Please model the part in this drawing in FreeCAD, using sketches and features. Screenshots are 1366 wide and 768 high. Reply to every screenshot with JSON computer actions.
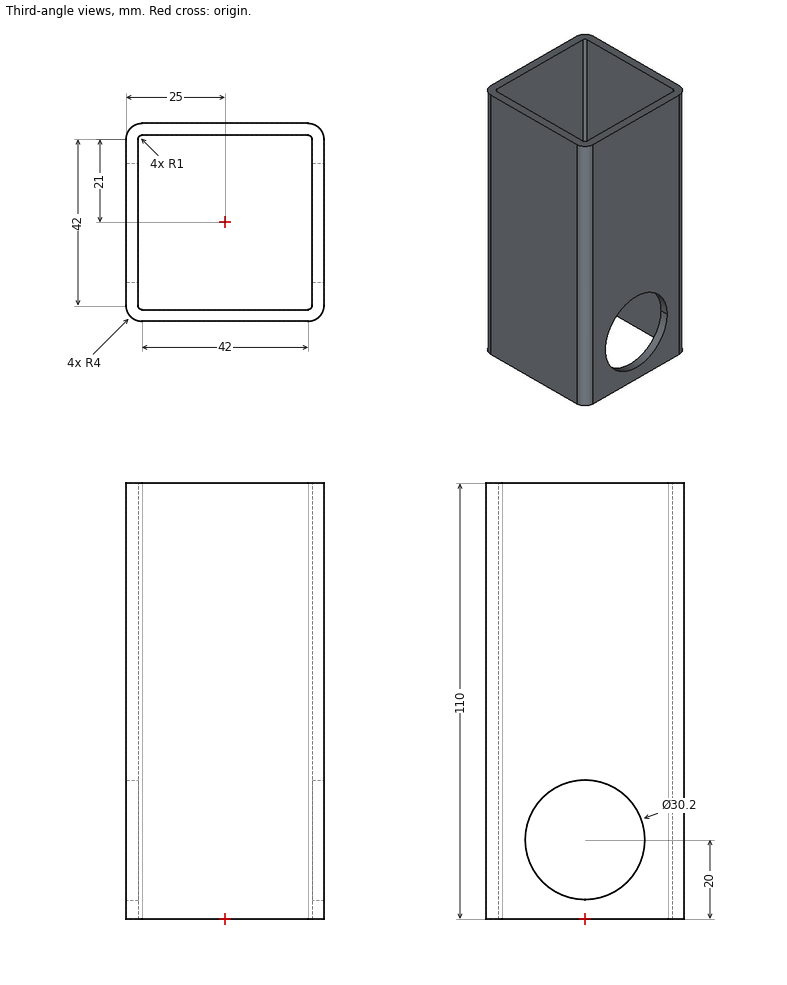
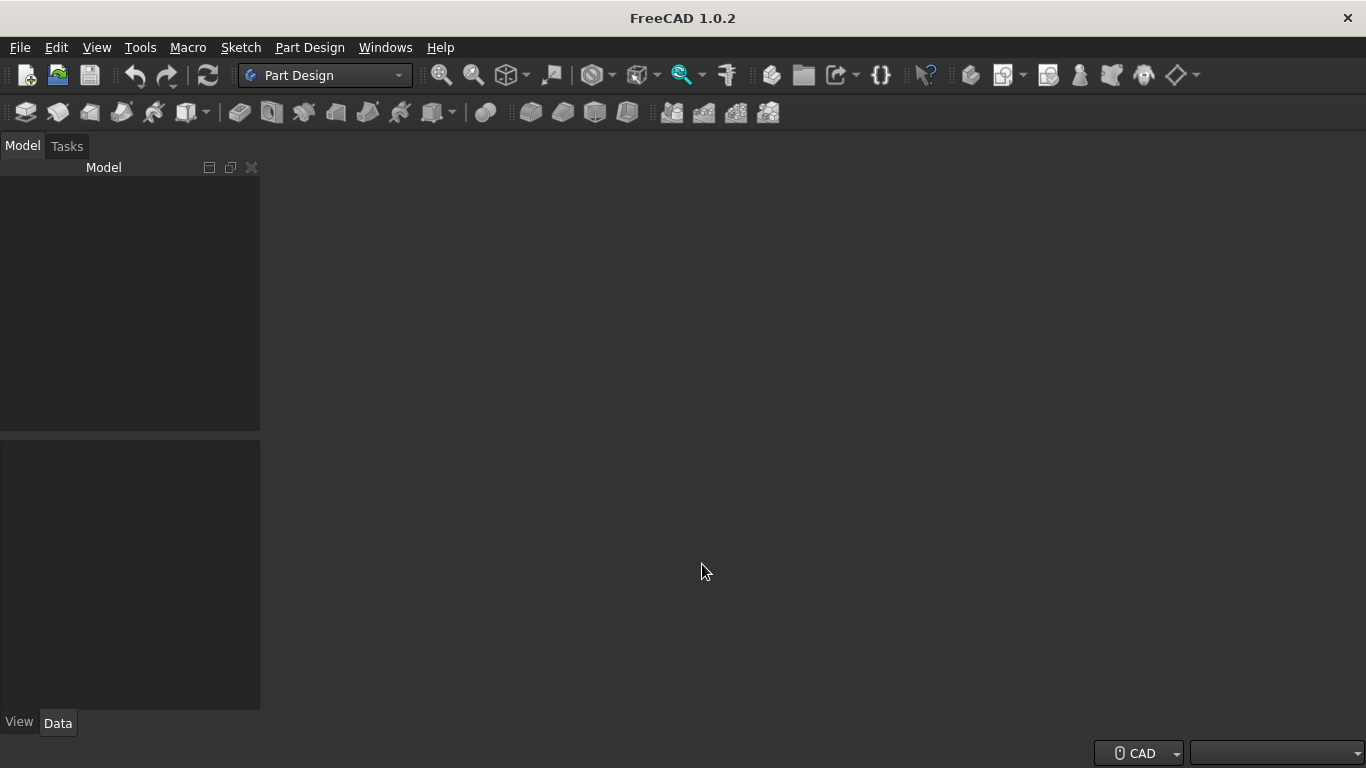
{"action": "left_click", "coordinate": [26, 76]}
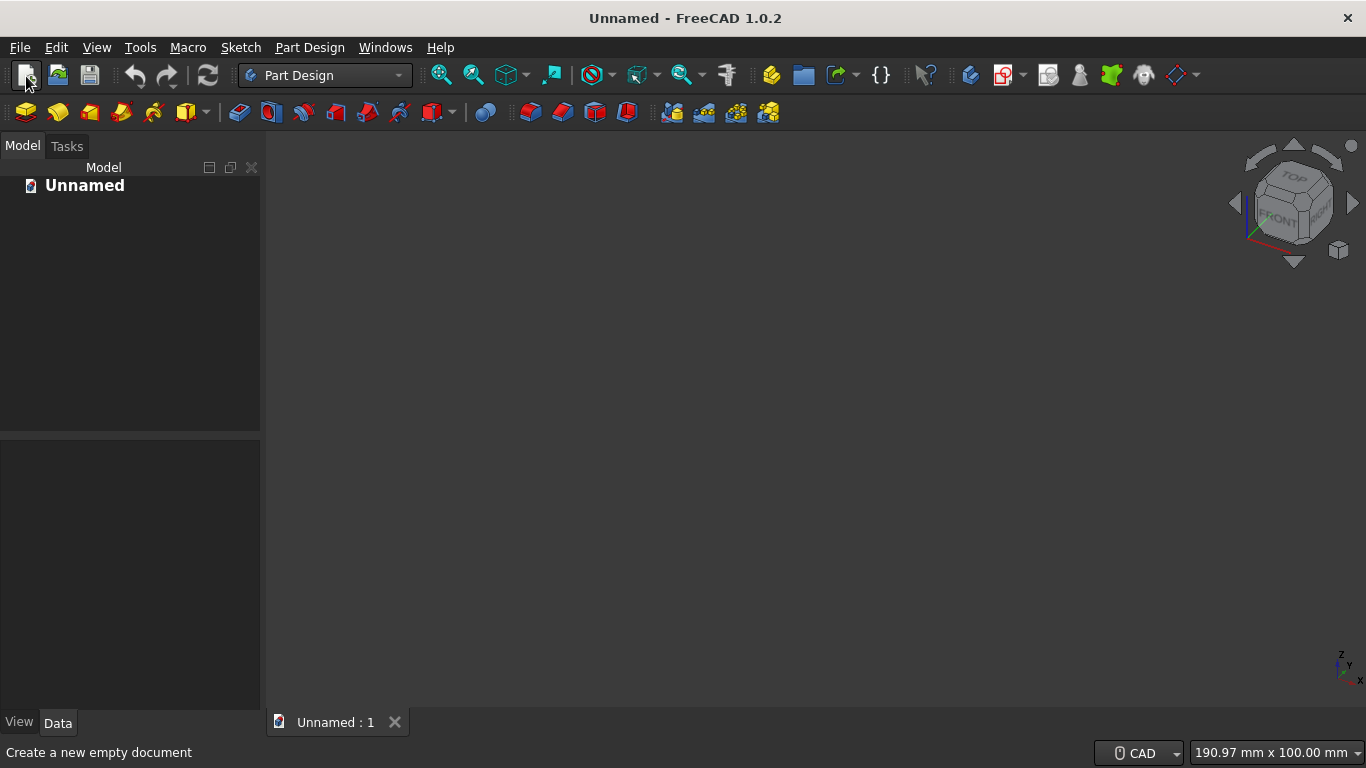
{"action": "left_click", "coordinate": [1004, 76]}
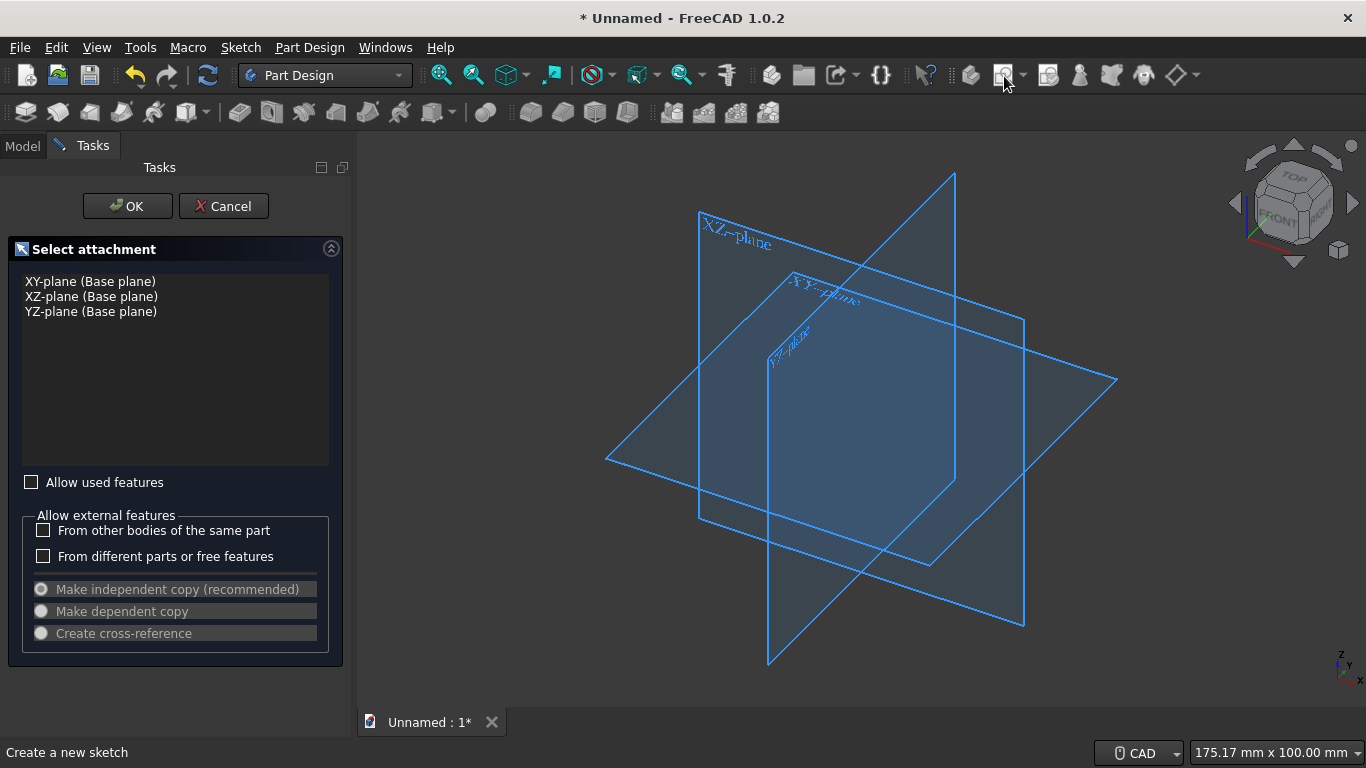
{"action": "left_click", "coordinate": [82, 282]}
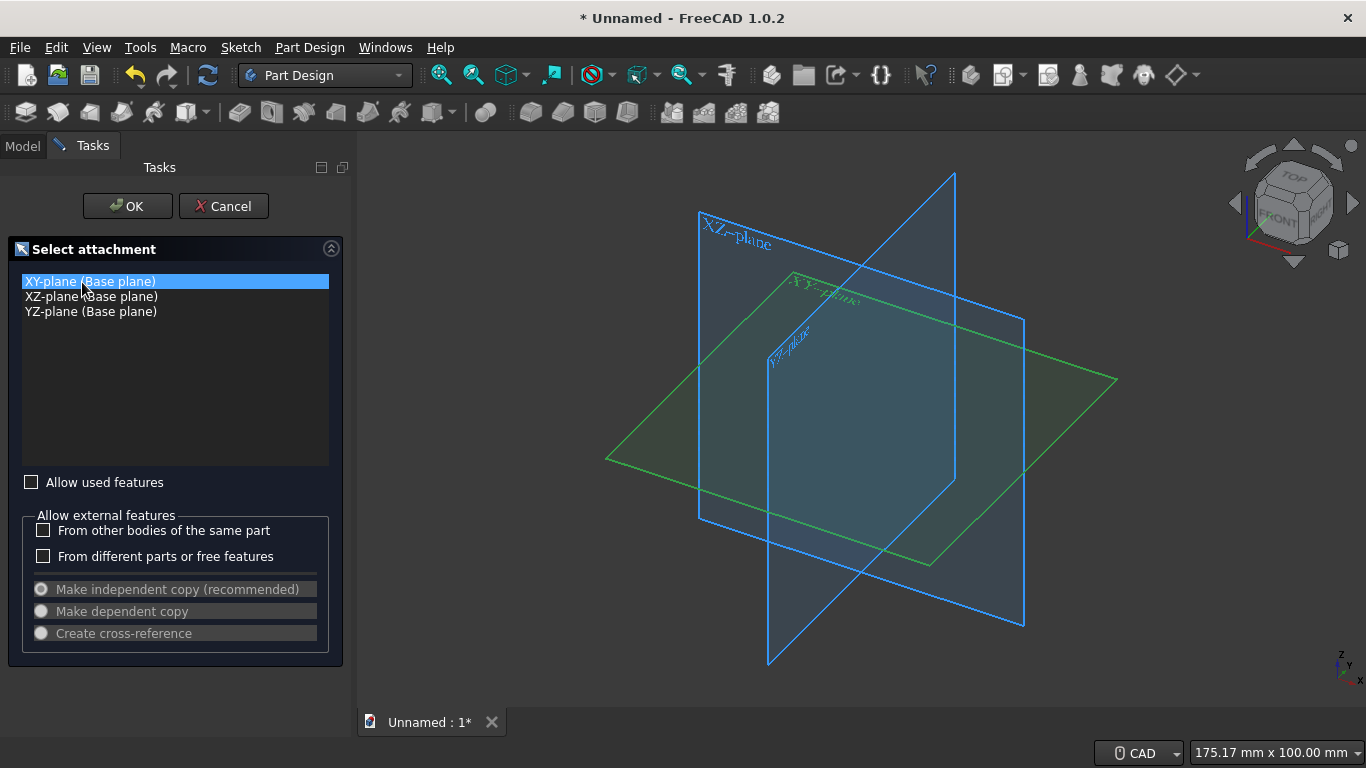
{"action": "left_click", "coordinate": [128, 206]}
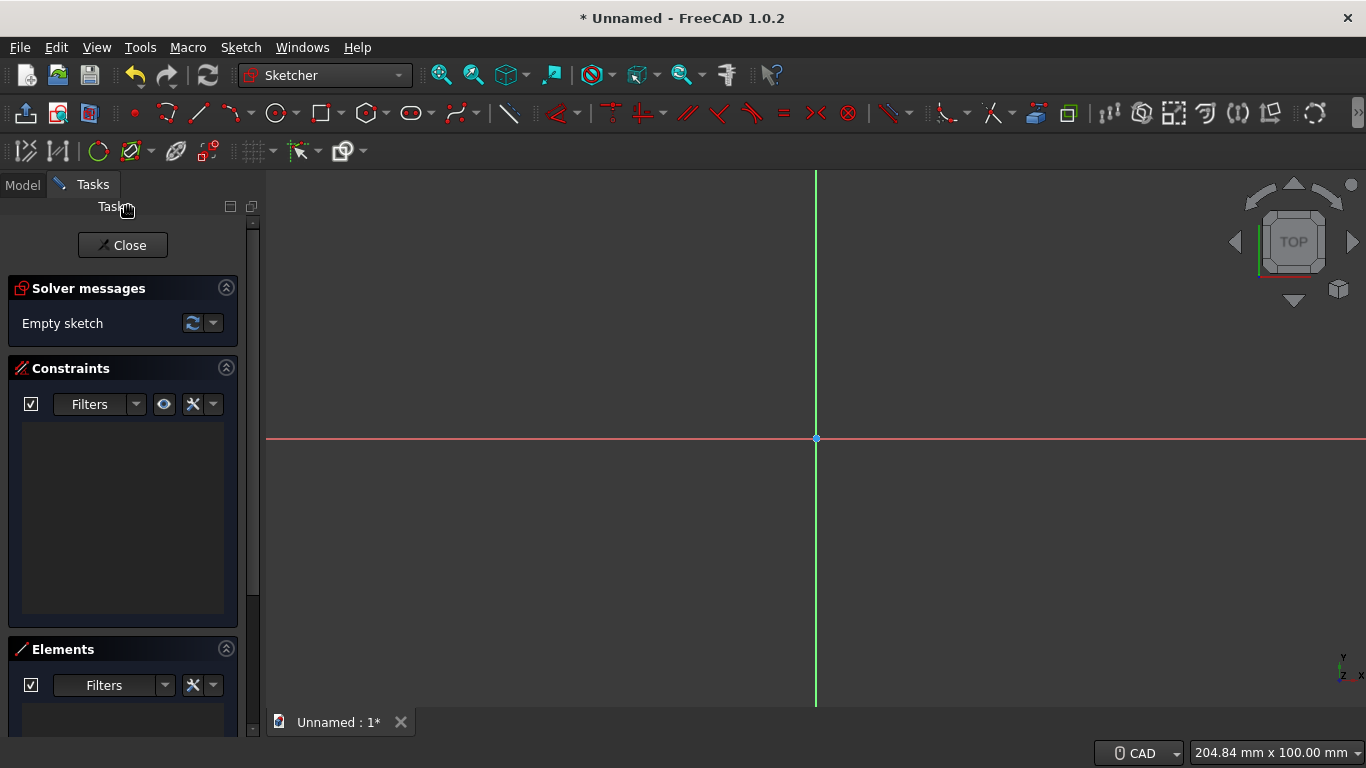
{"action": "left_click", "coordinate": [200, 114]}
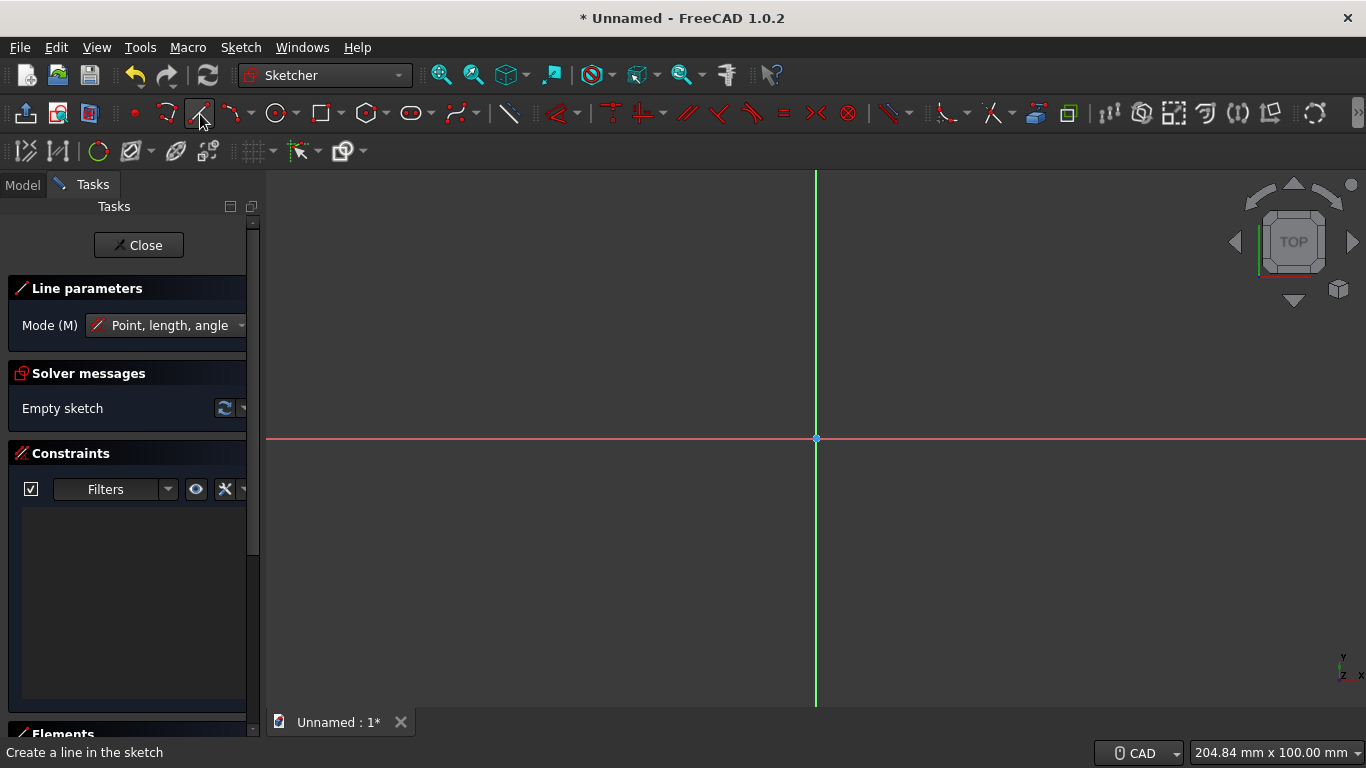
{"action": "left_click", "coordinate": [682, 326]}
{"action": "left_click", "coordinate": [682, 551]}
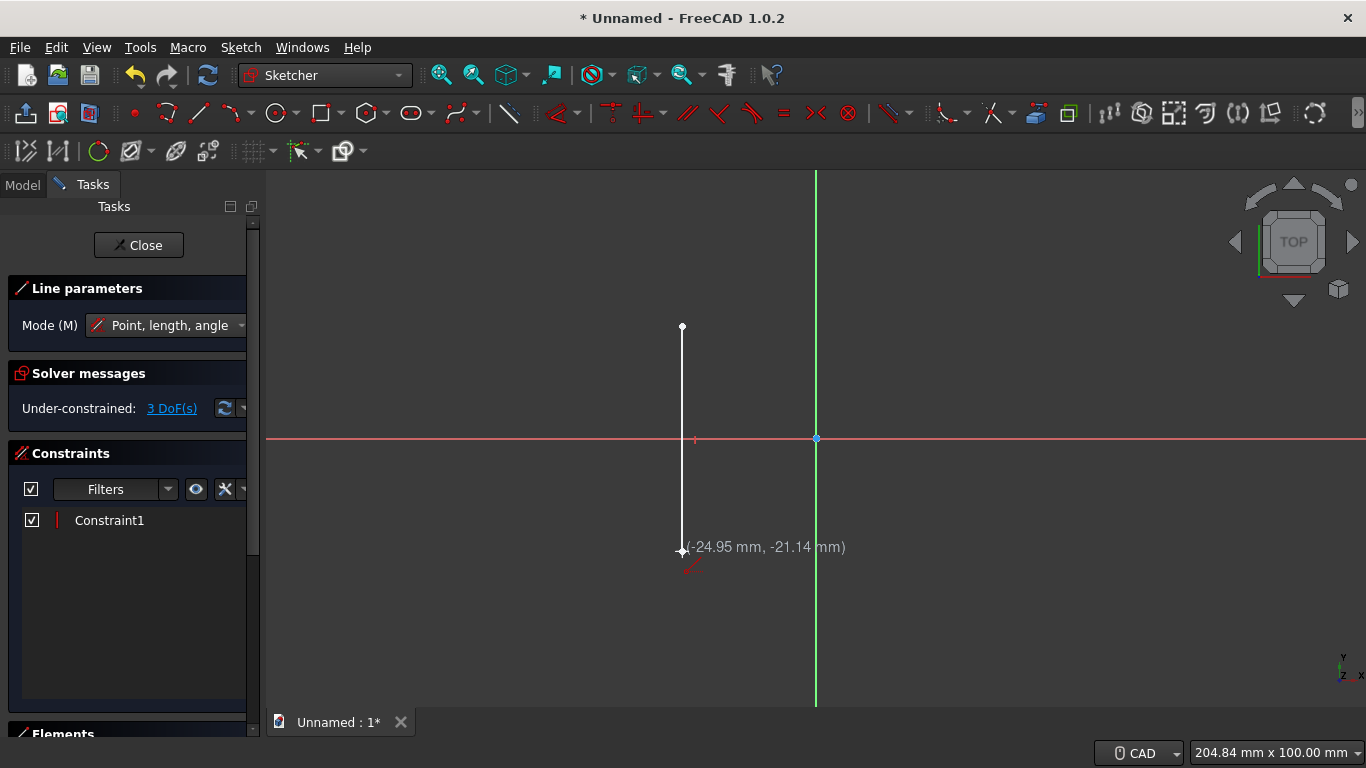
{"action": "left_click", "coordinate": [703, 573]}
{"action": "left_click", "coordinate": [929, 573]}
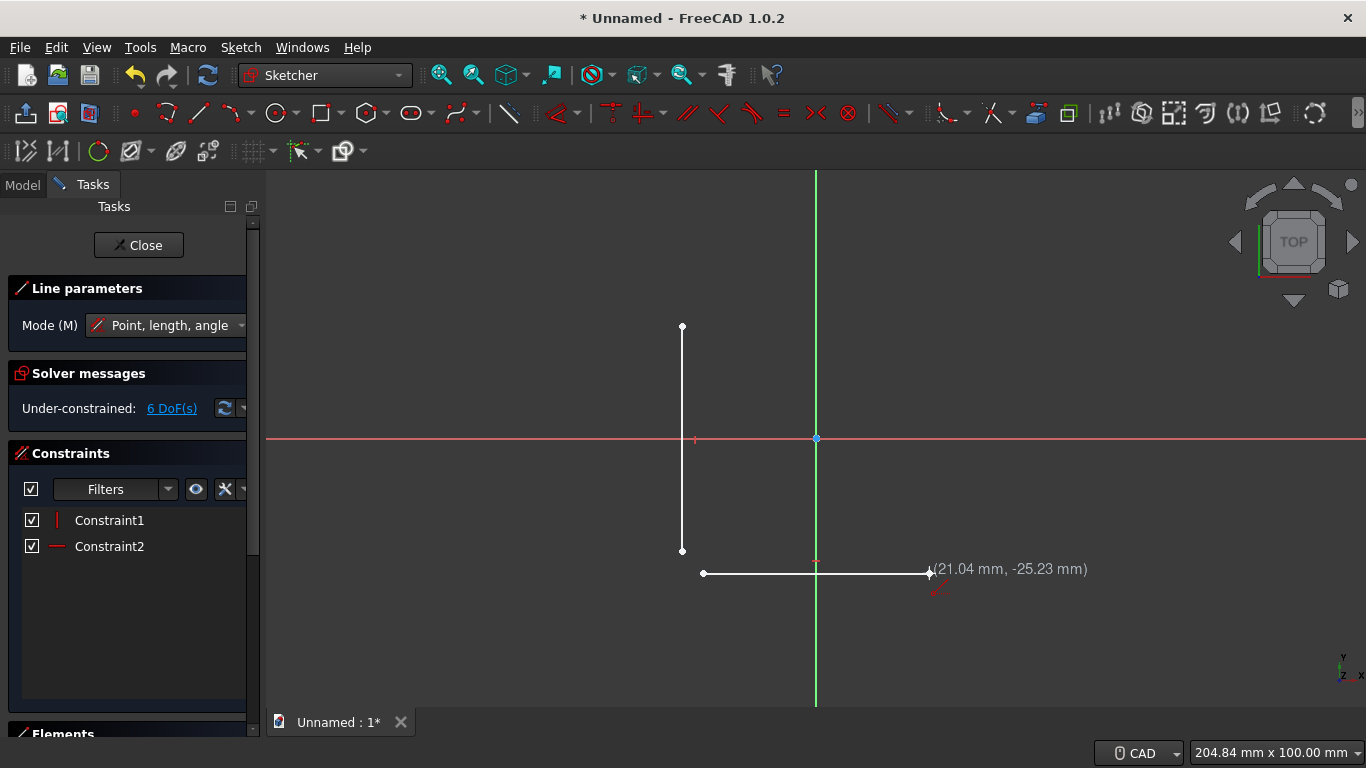
{"action": "left_click", "coordinate": [950, 551]}
{"action": "left_click", "coordinate": [950, 326]}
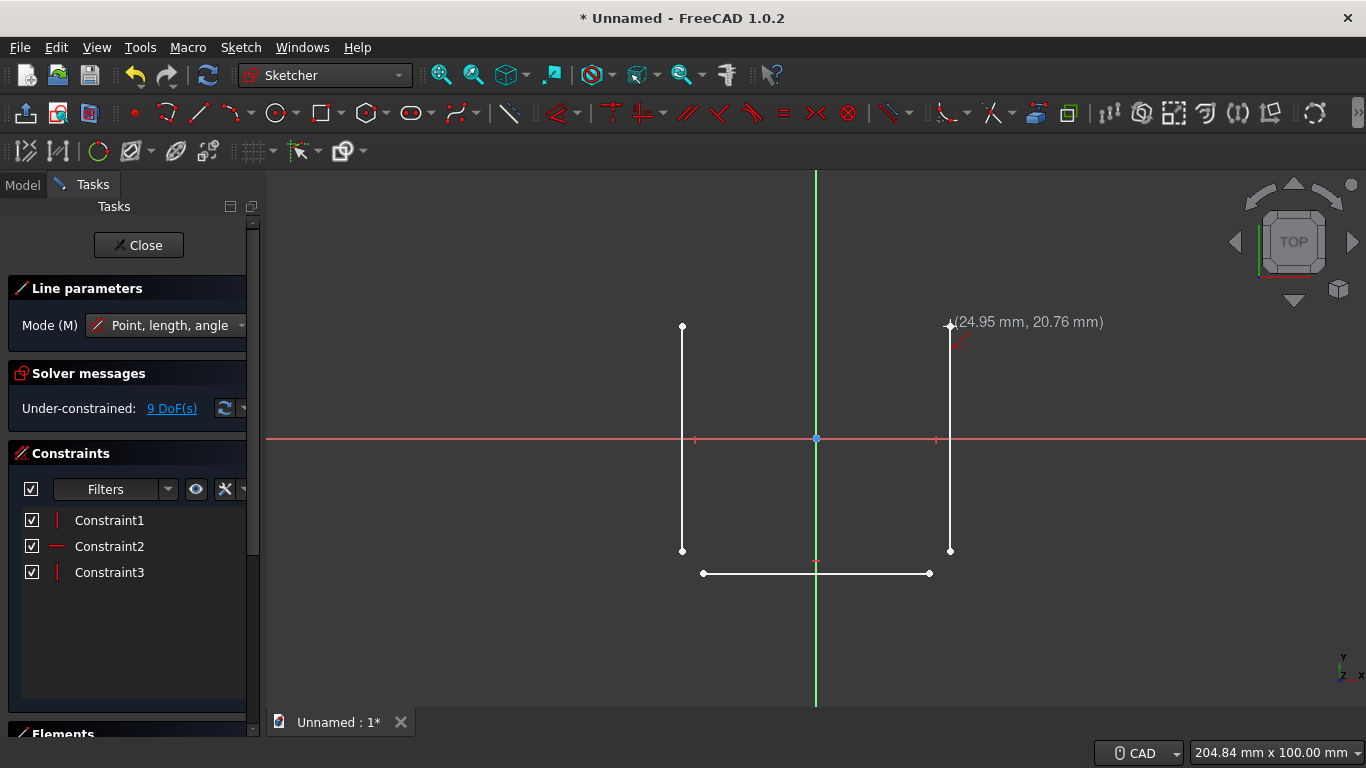
{"action": "left_click", "coordinate": [929, 304]}
{"action": "left_click", "coordinate": [703, 304]}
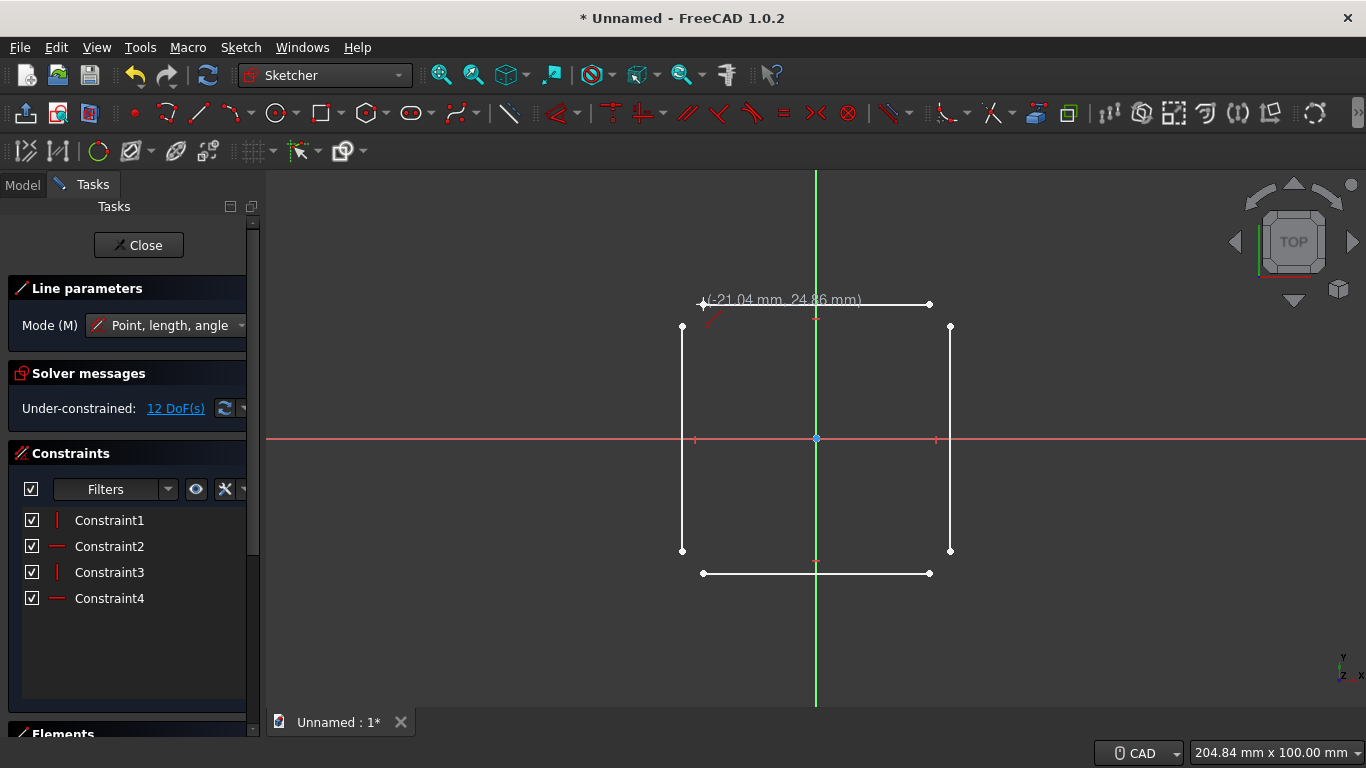
{"action": "left_click", "coordinate": [232, 114]}